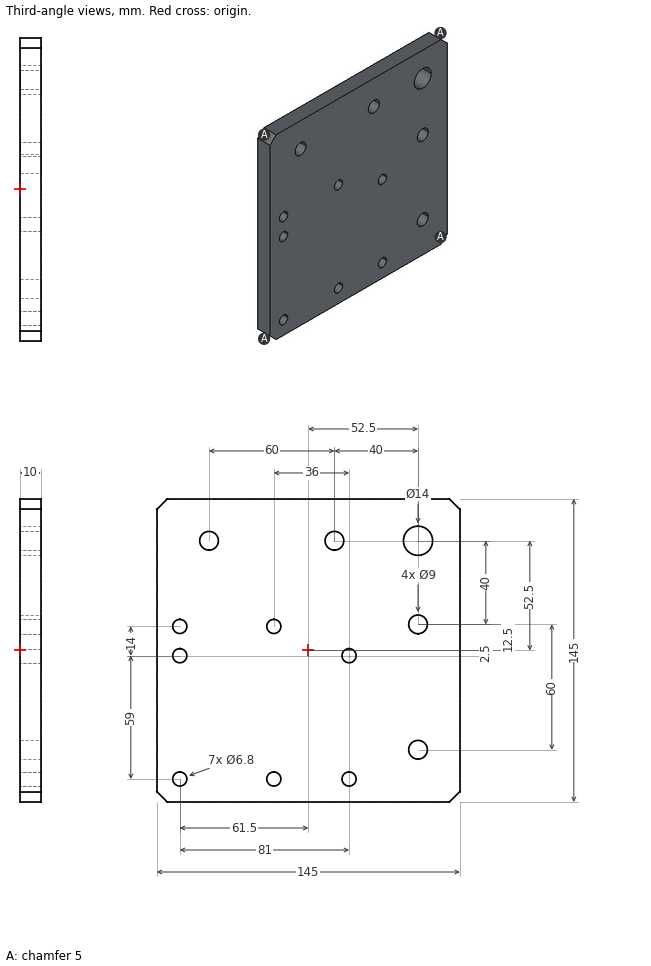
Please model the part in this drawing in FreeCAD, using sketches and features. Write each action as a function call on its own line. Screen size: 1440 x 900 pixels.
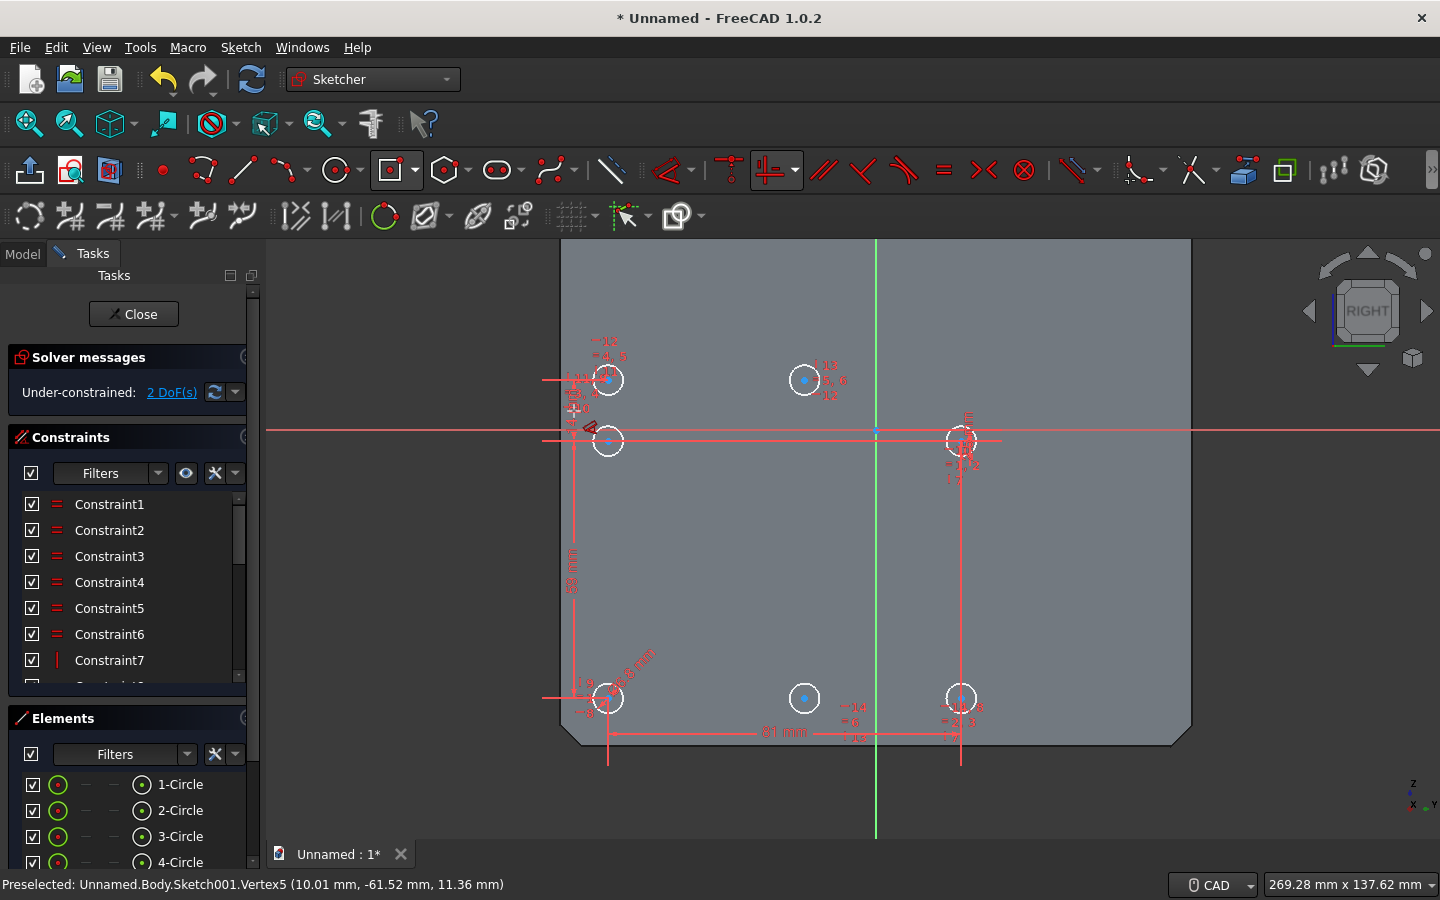
click(961, 441)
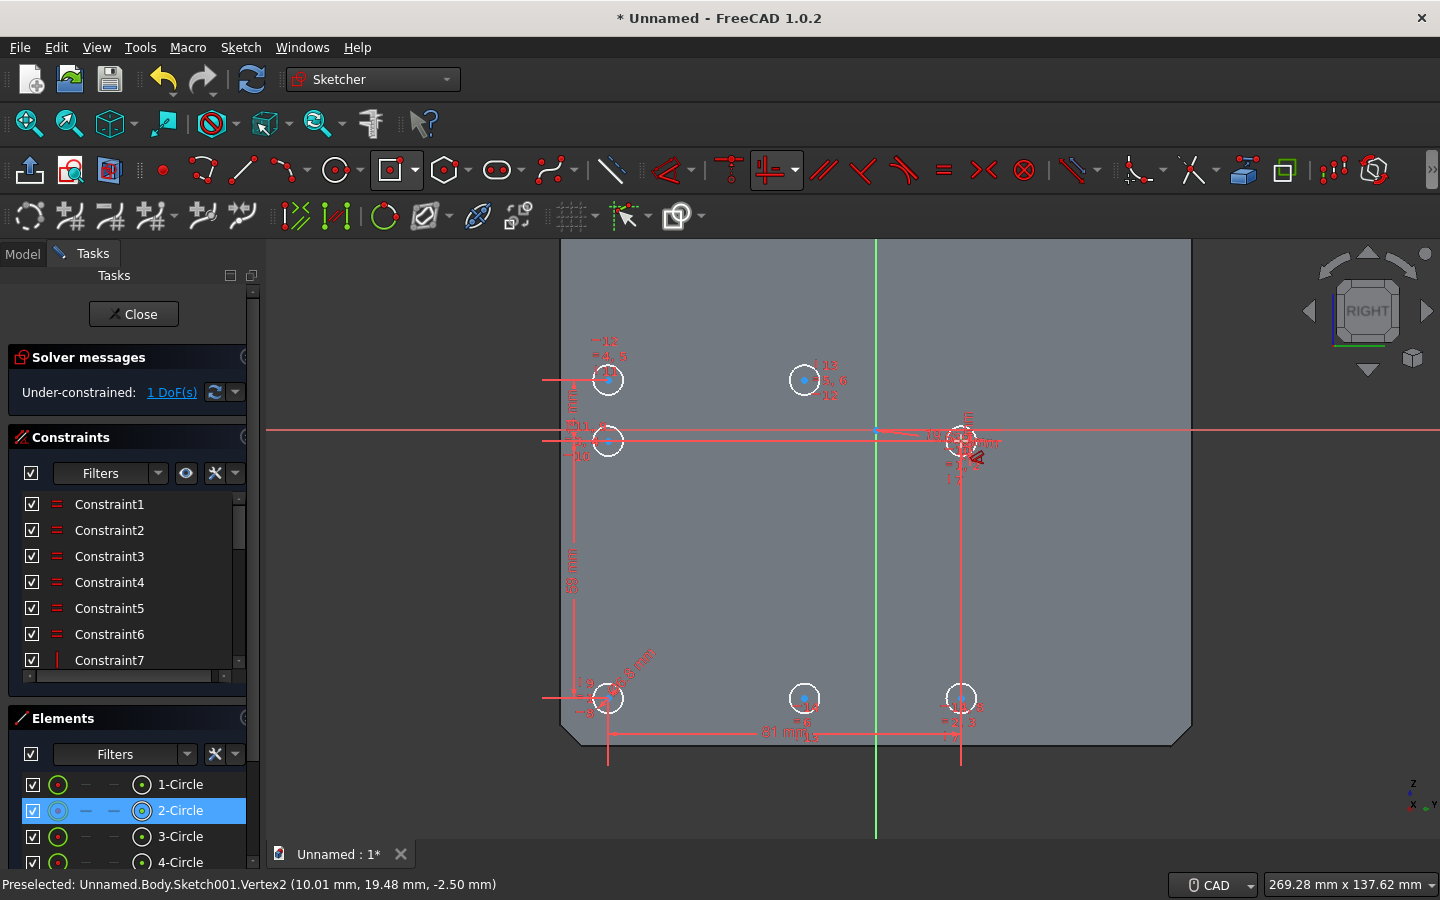
click(805, 380)
click(847, 346)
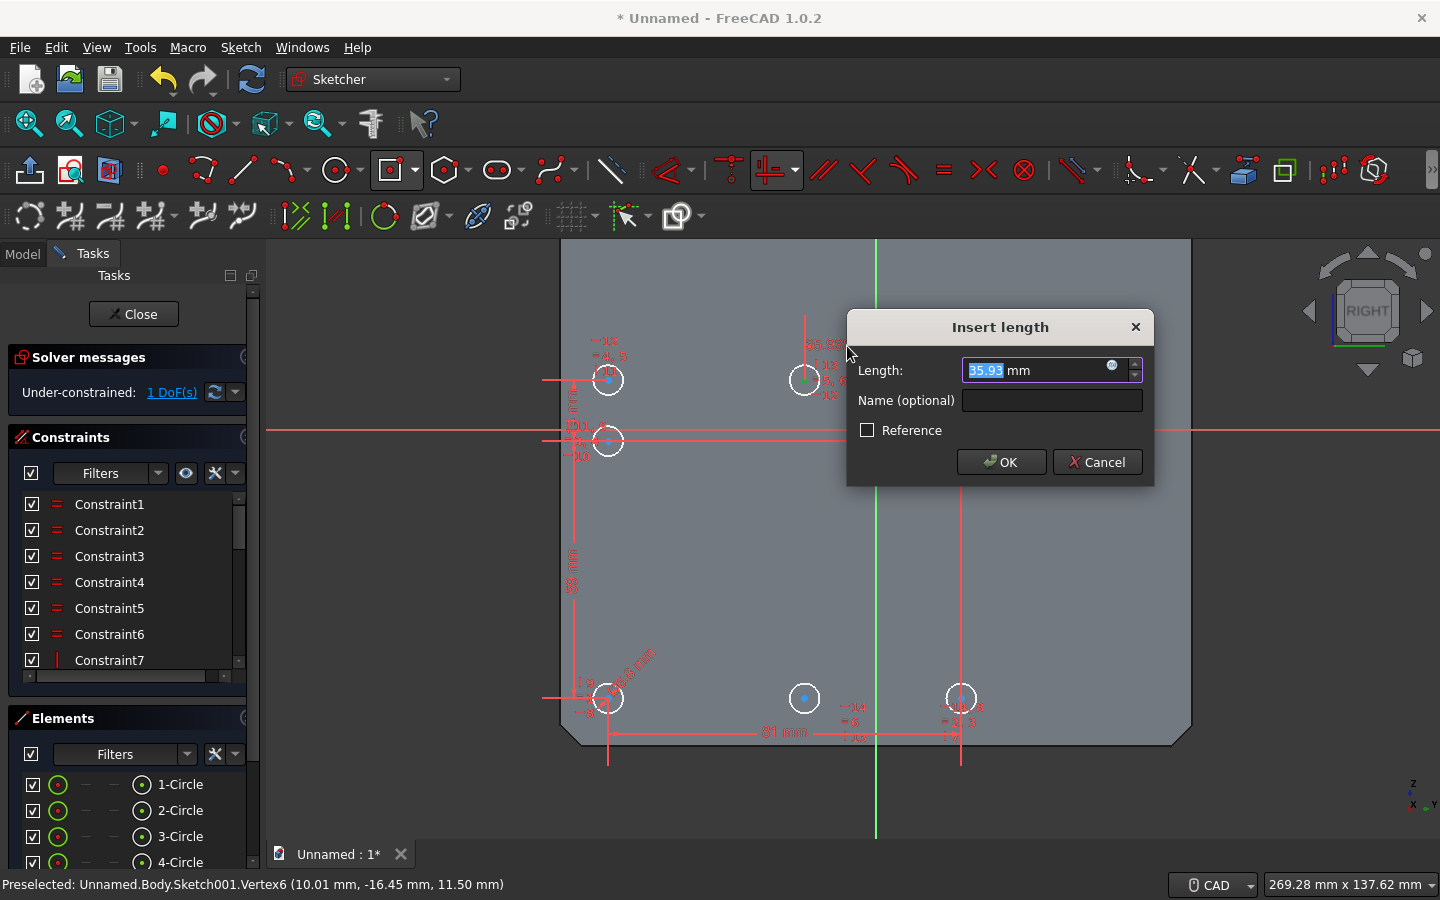
text(36)
key(Return)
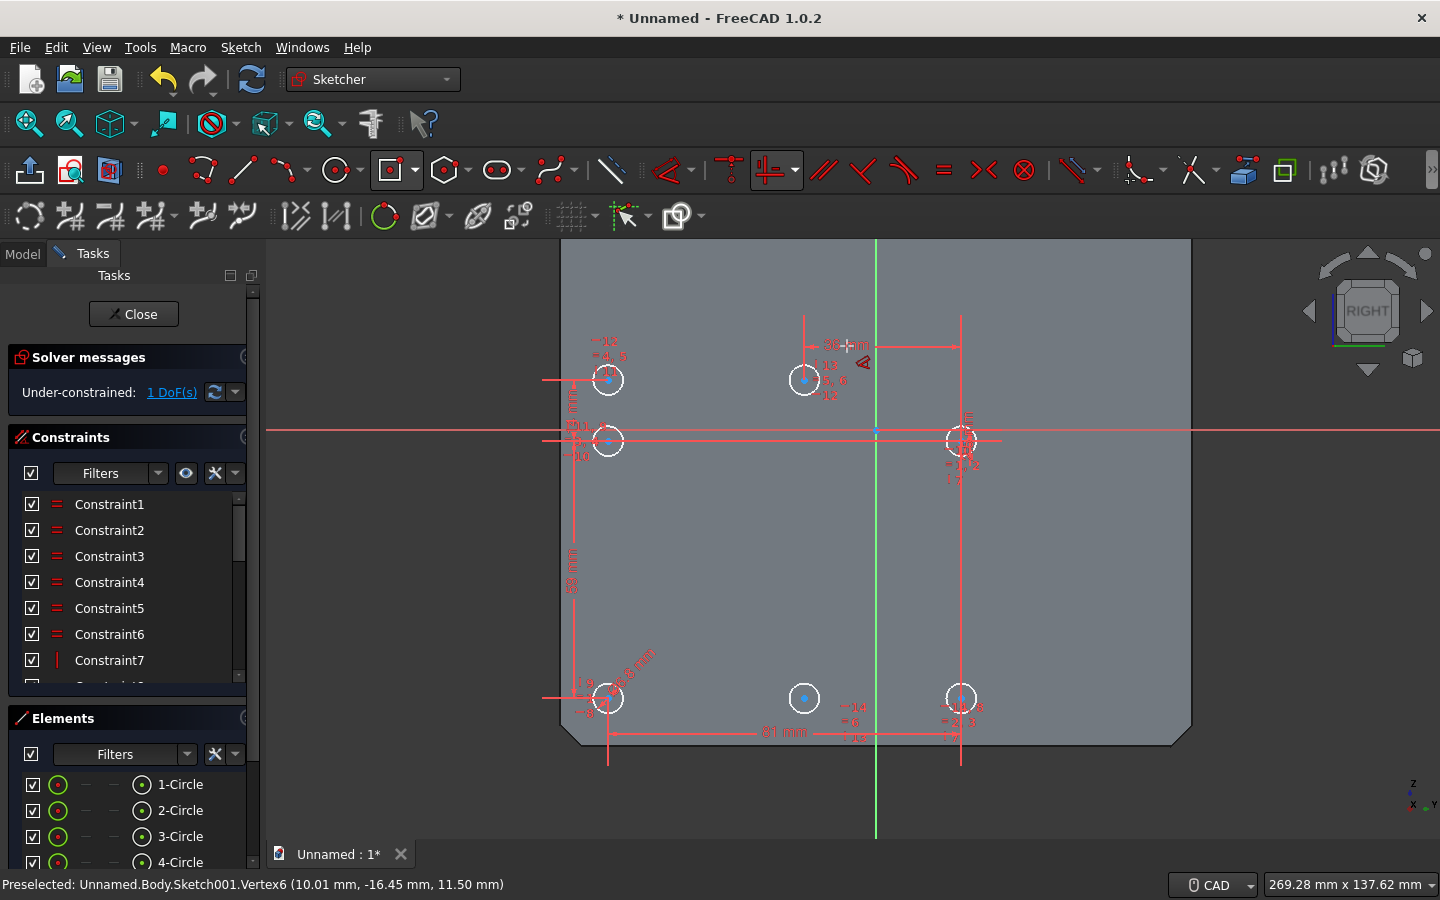
click(608, 698)
click(681, 732)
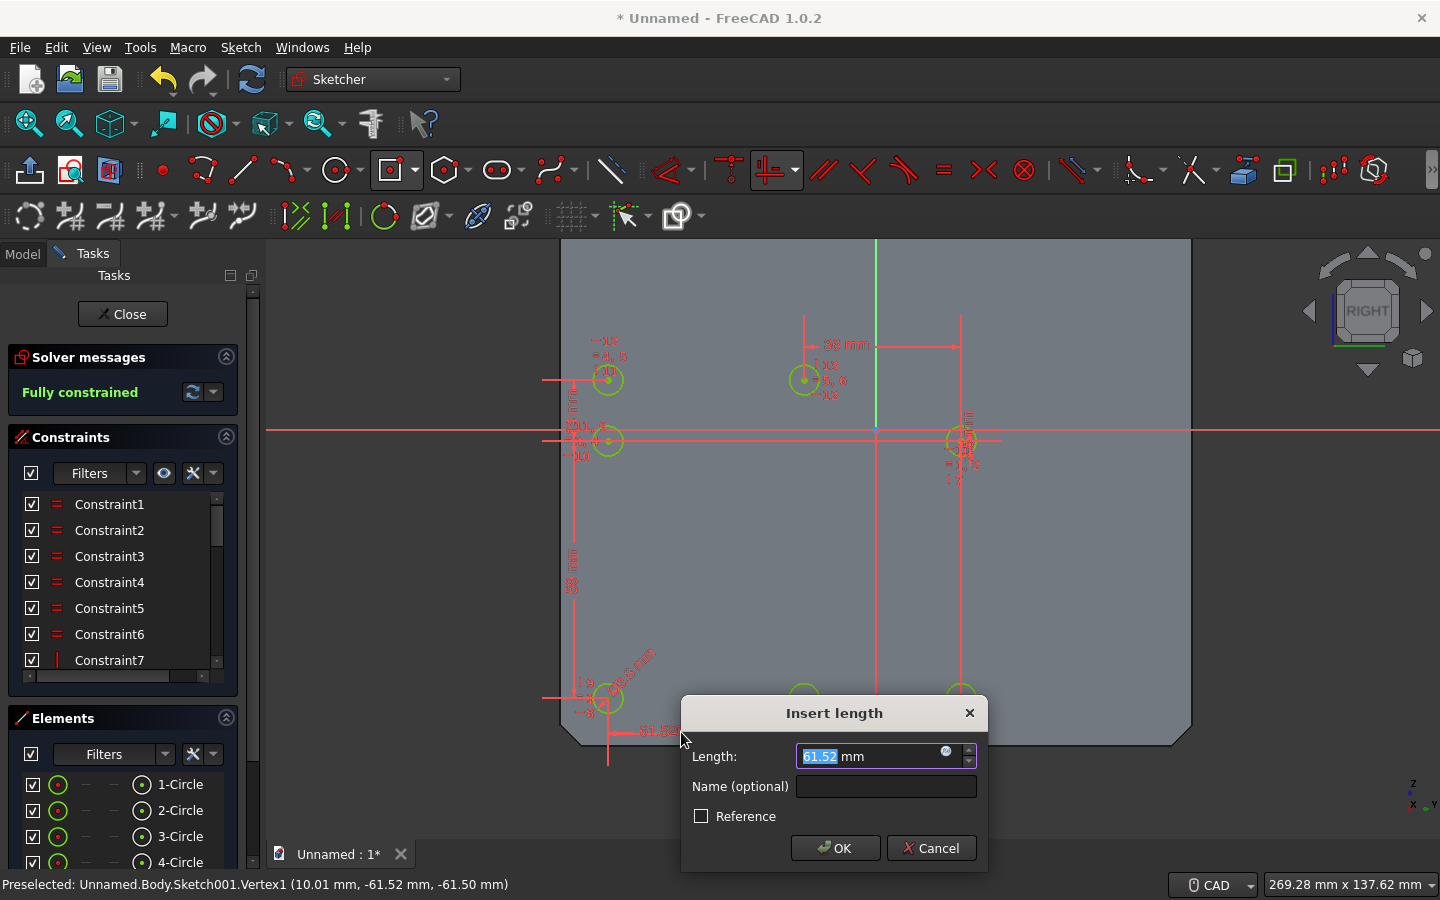
text(61.5)
key(Return)
key(Escape)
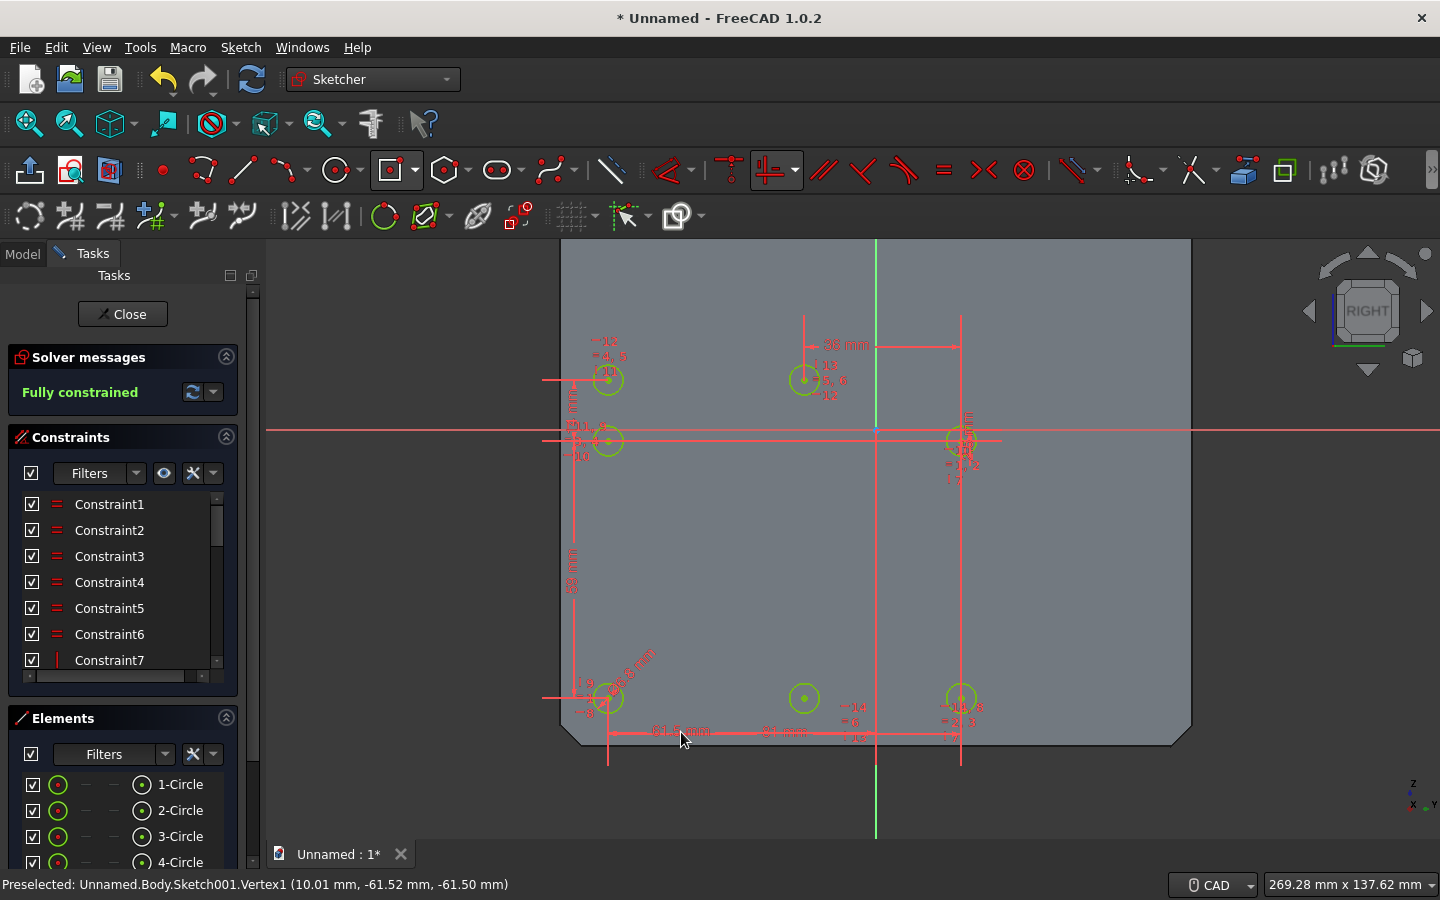
click(123, 314)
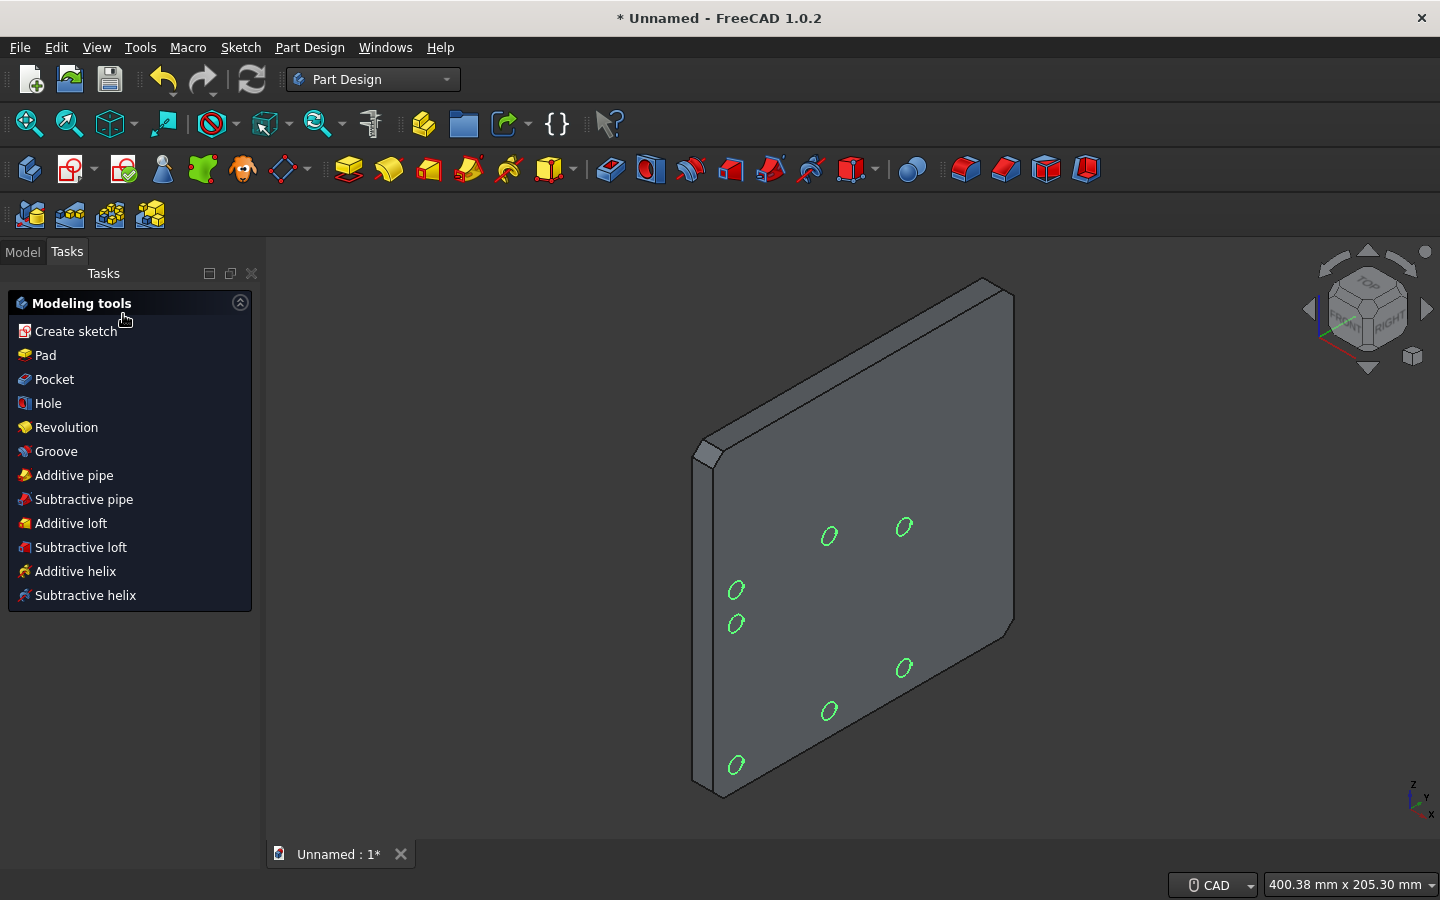
click(612, 170)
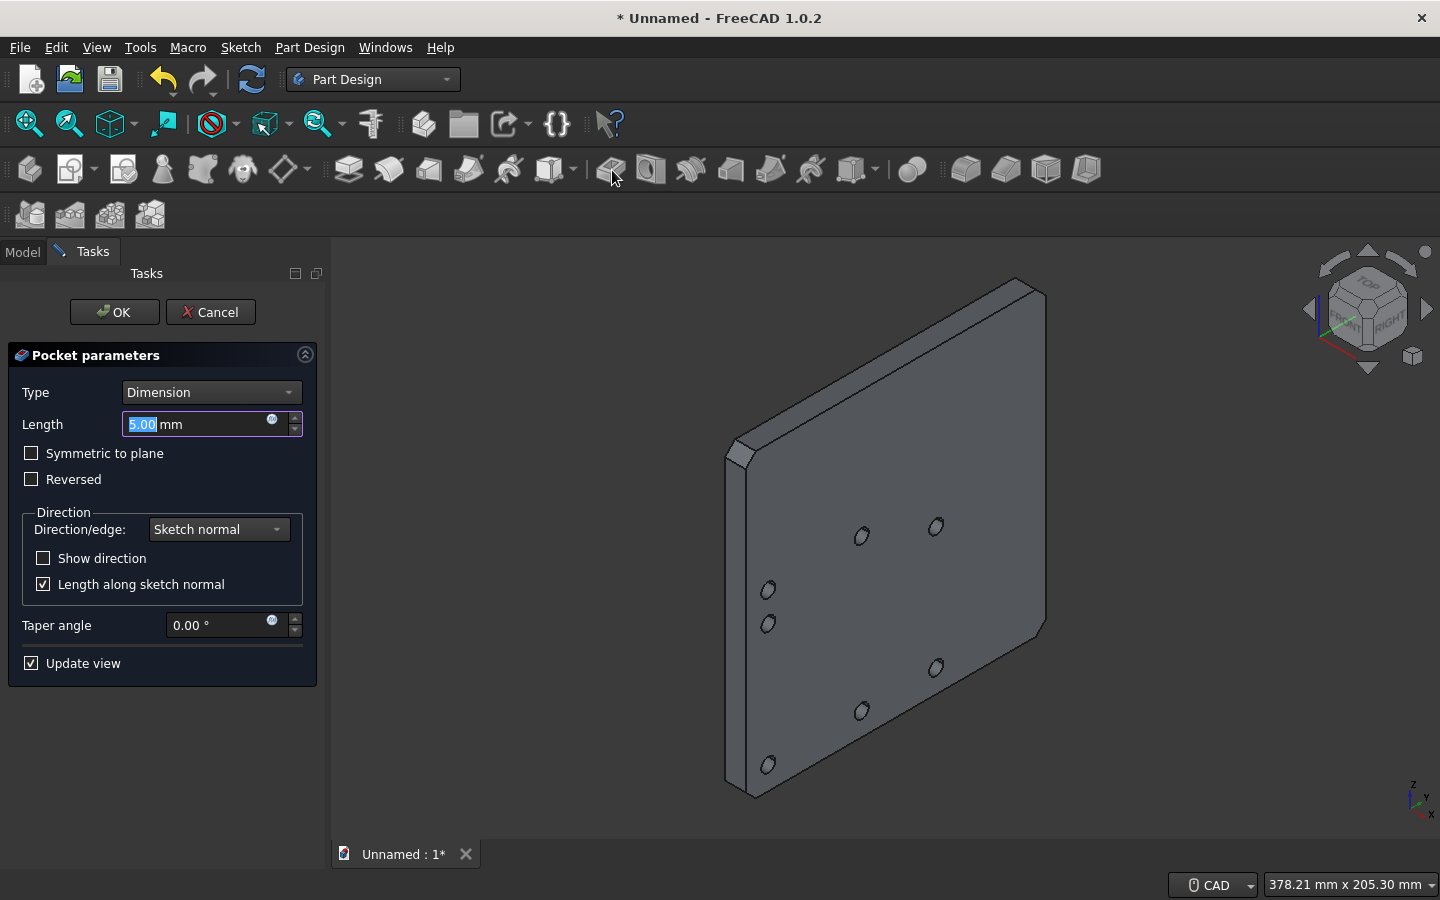
click(212, 392)